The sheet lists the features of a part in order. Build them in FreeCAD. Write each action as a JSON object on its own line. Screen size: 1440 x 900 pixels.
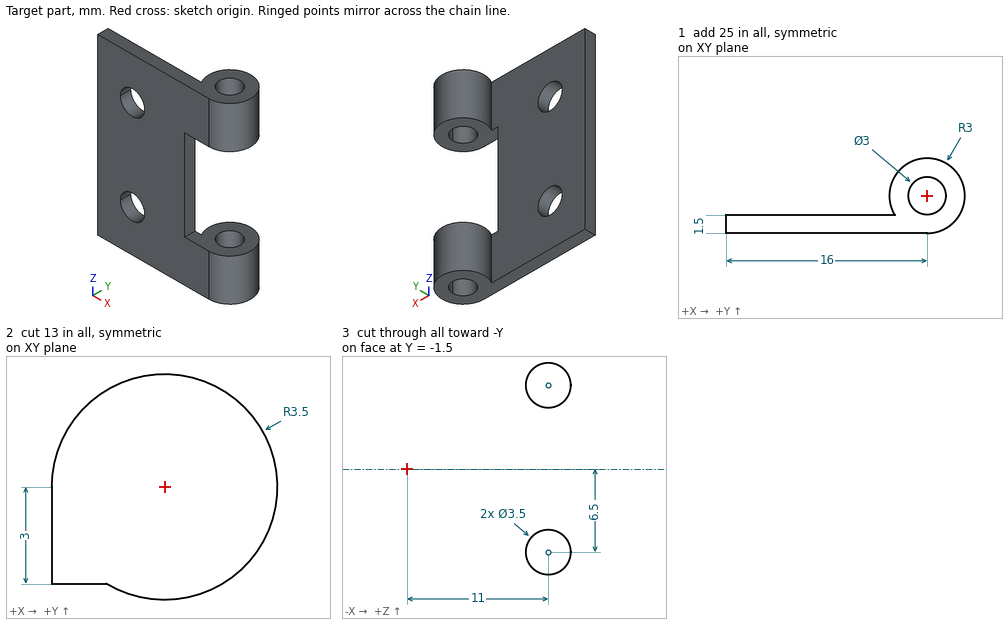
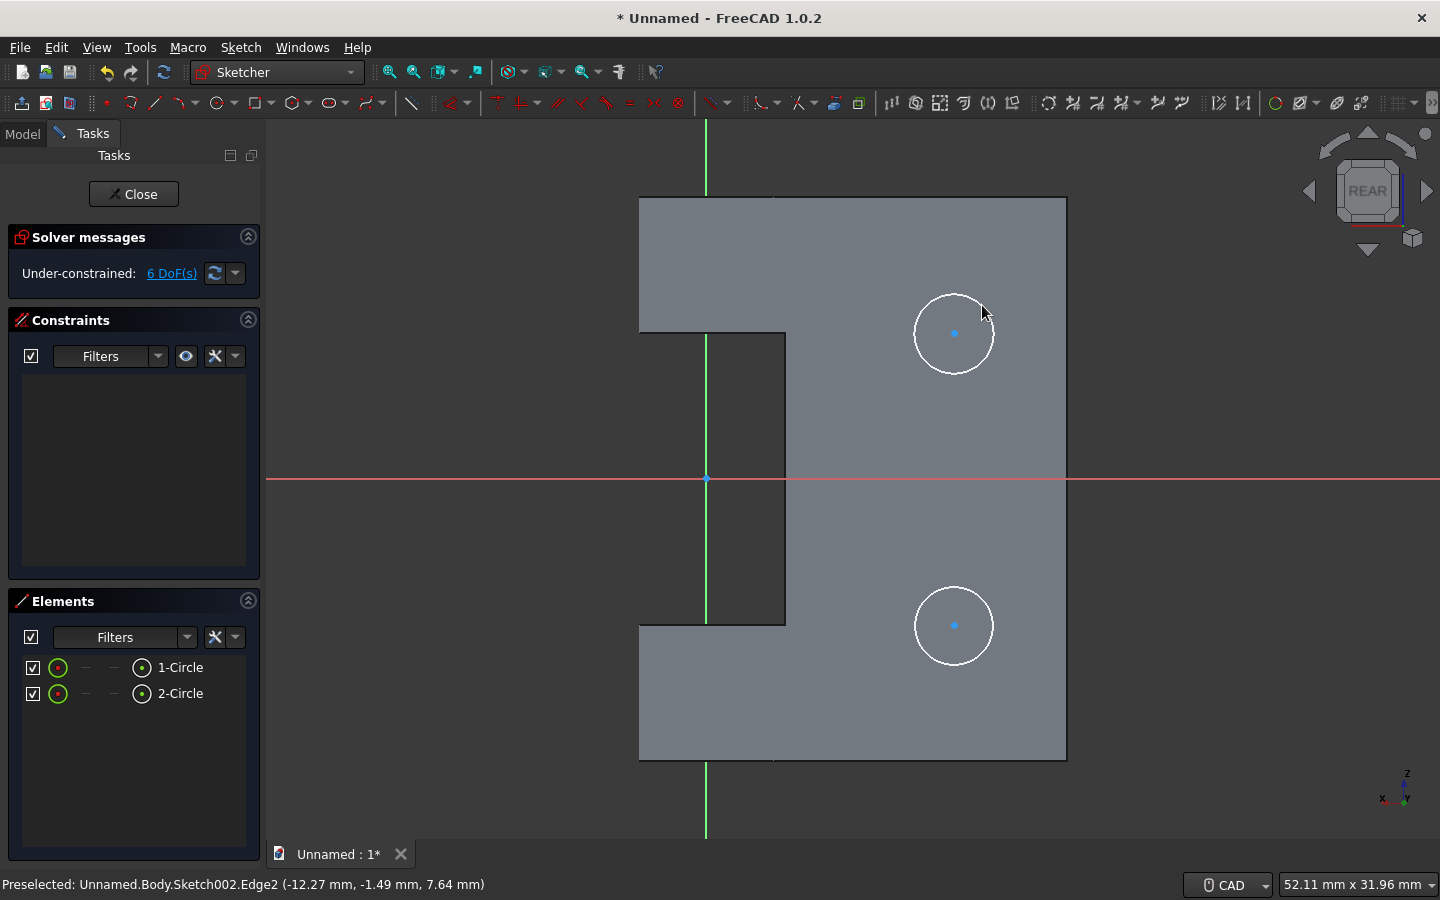
{"action": "left_click", "coordinate": [981, 598]}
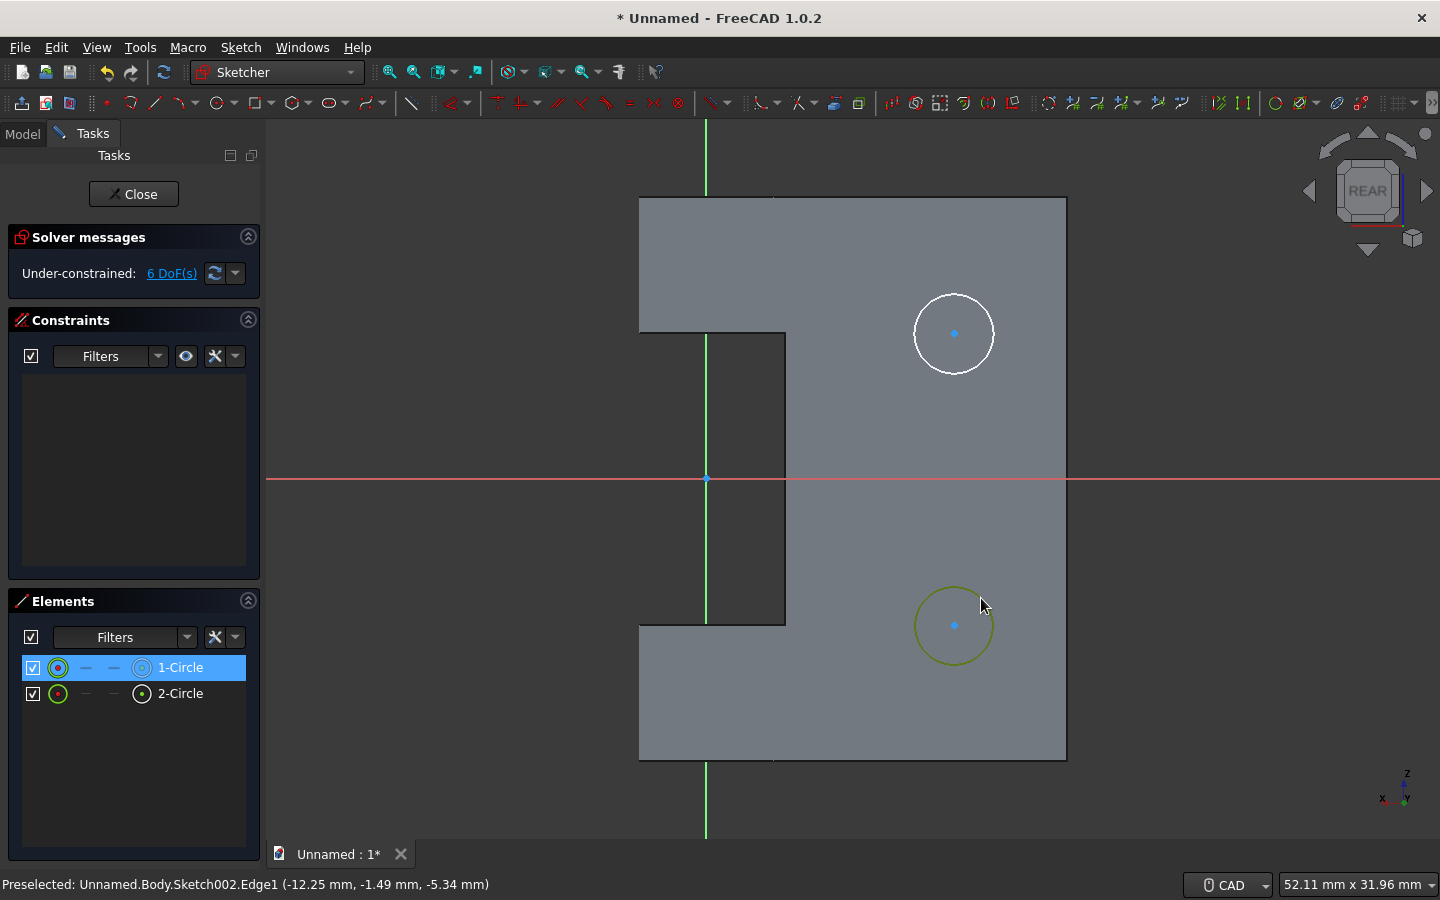
{"action": "left_click", "coordinate": [982, 306]}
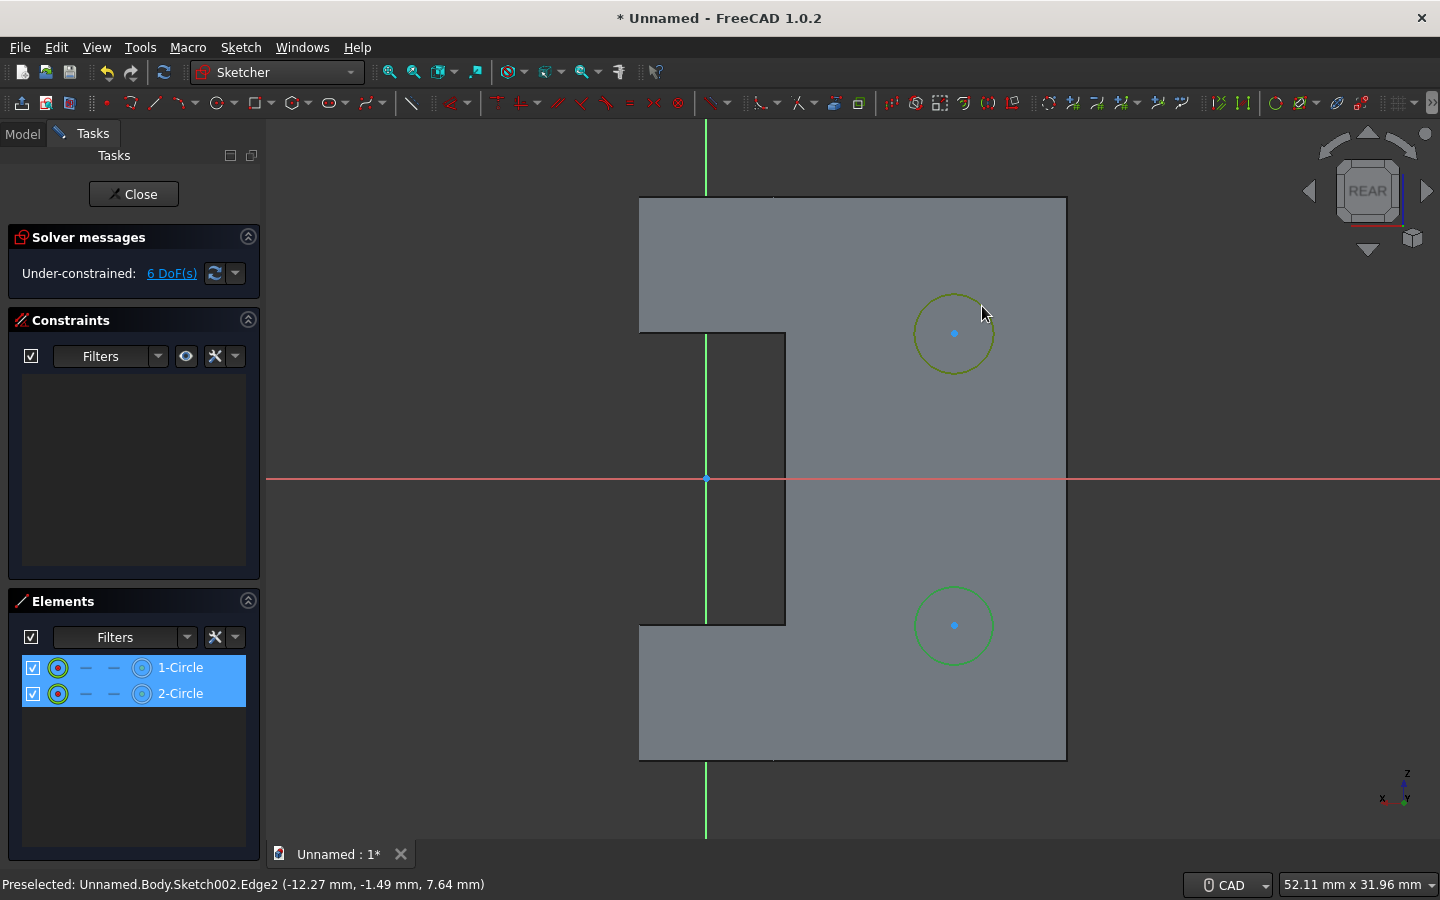
{"action": "left_click", "coordinate": [630, 104]}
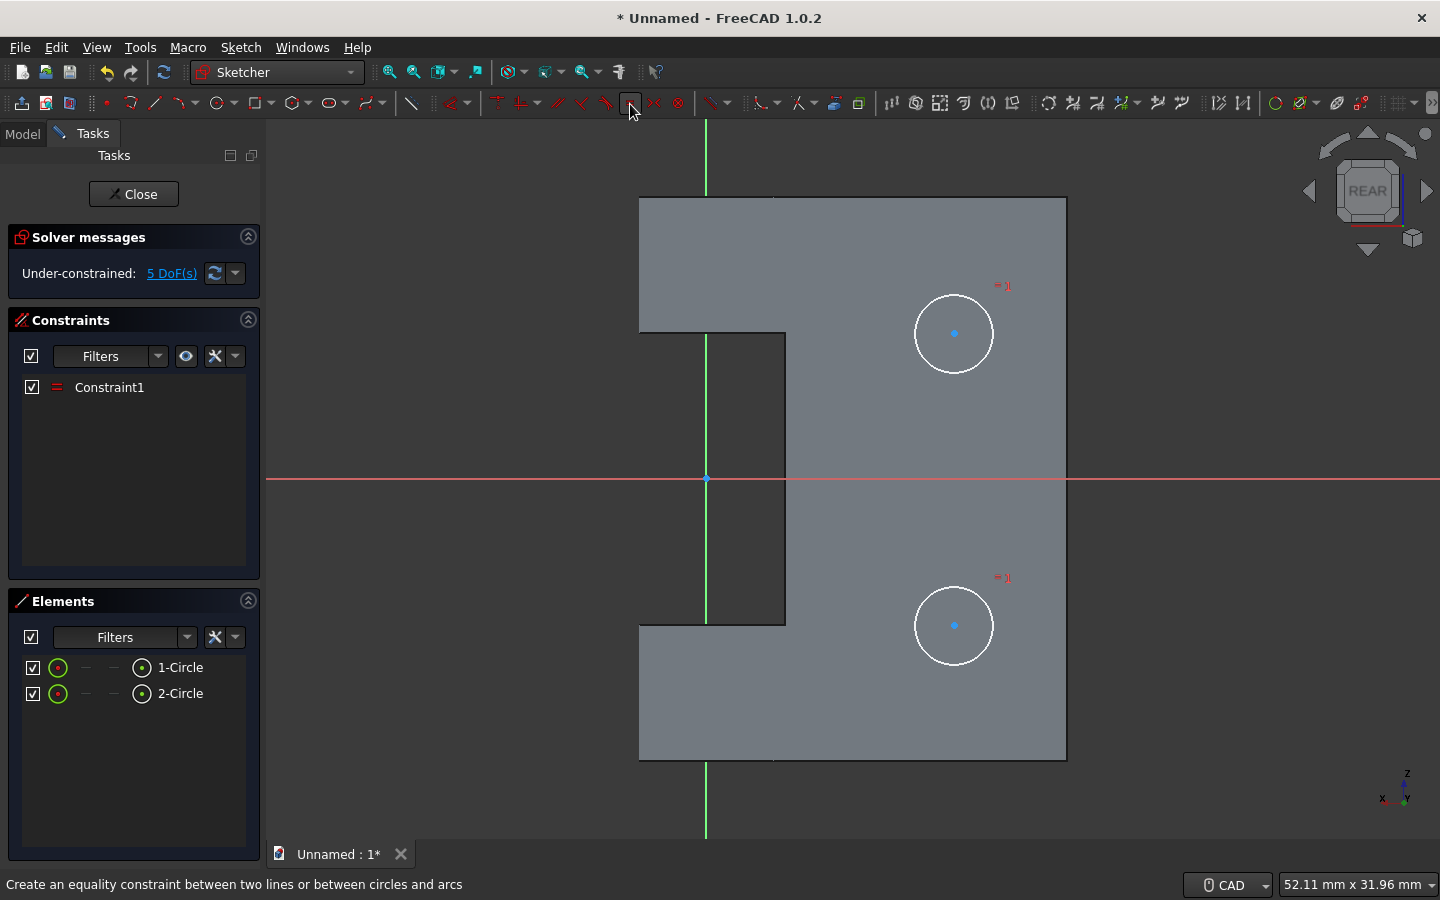
{"action": "left_click", "coordinate": [954, 626]}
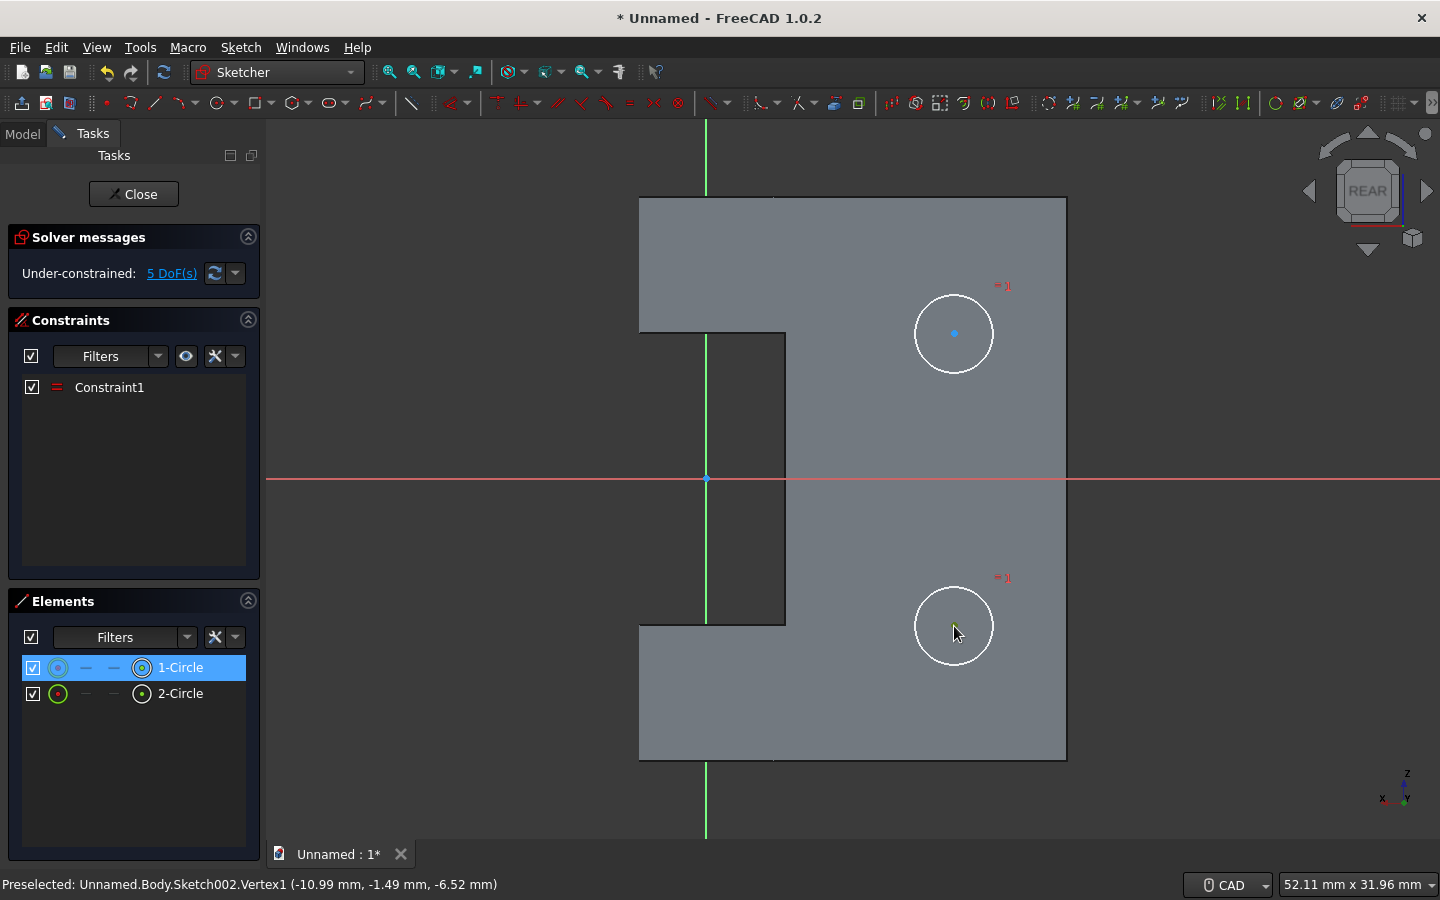
{"action": "left_click", "coordinate": [954, 334]}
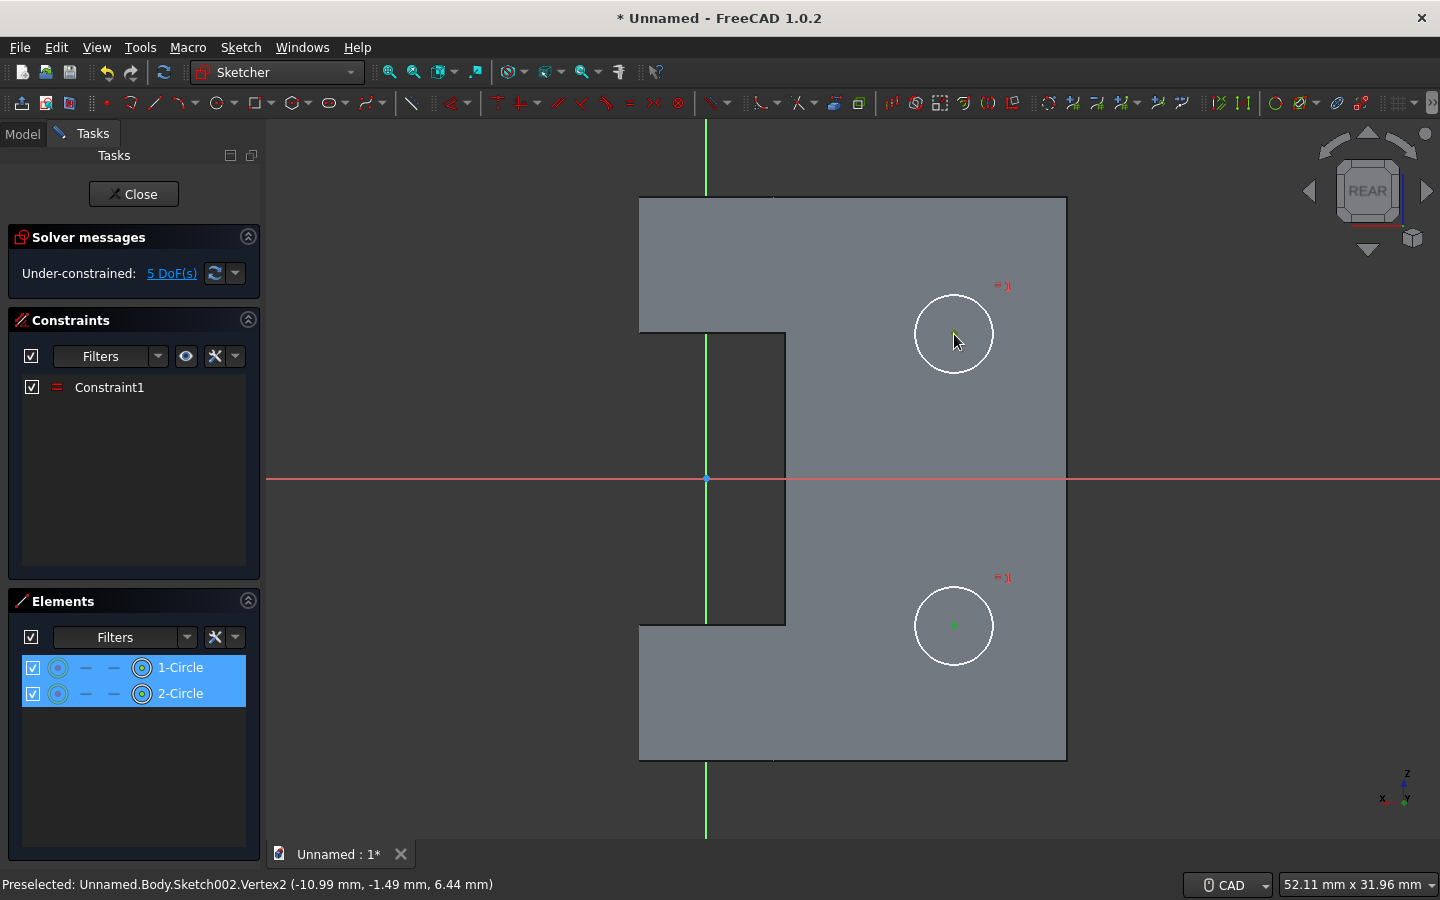
{"action": "left_click", "coordinate": [364, 479]}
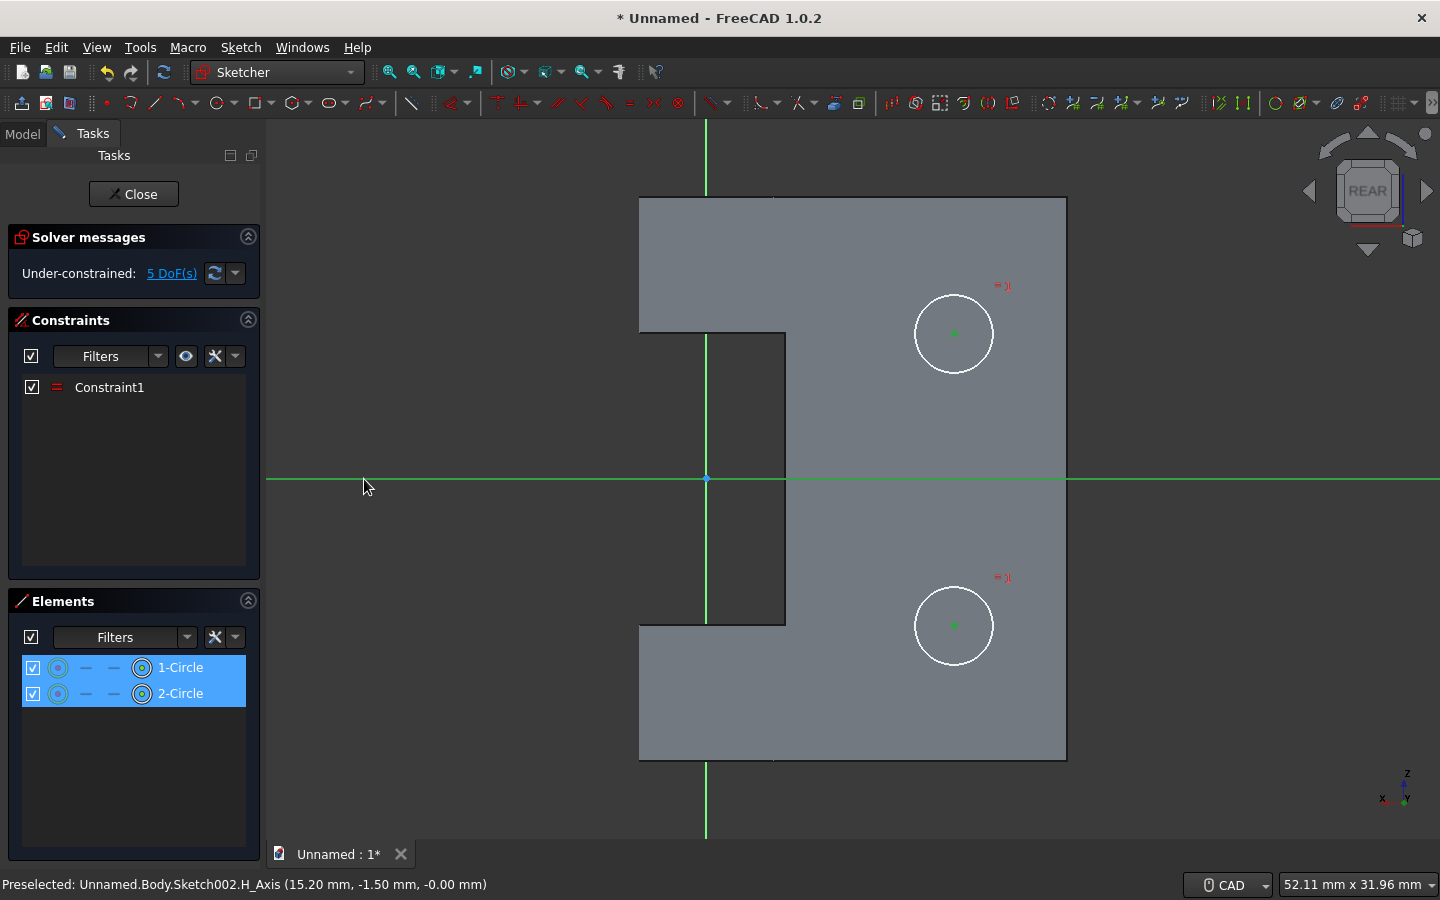
{"action": "left_click", "coordinate": [654, 104]}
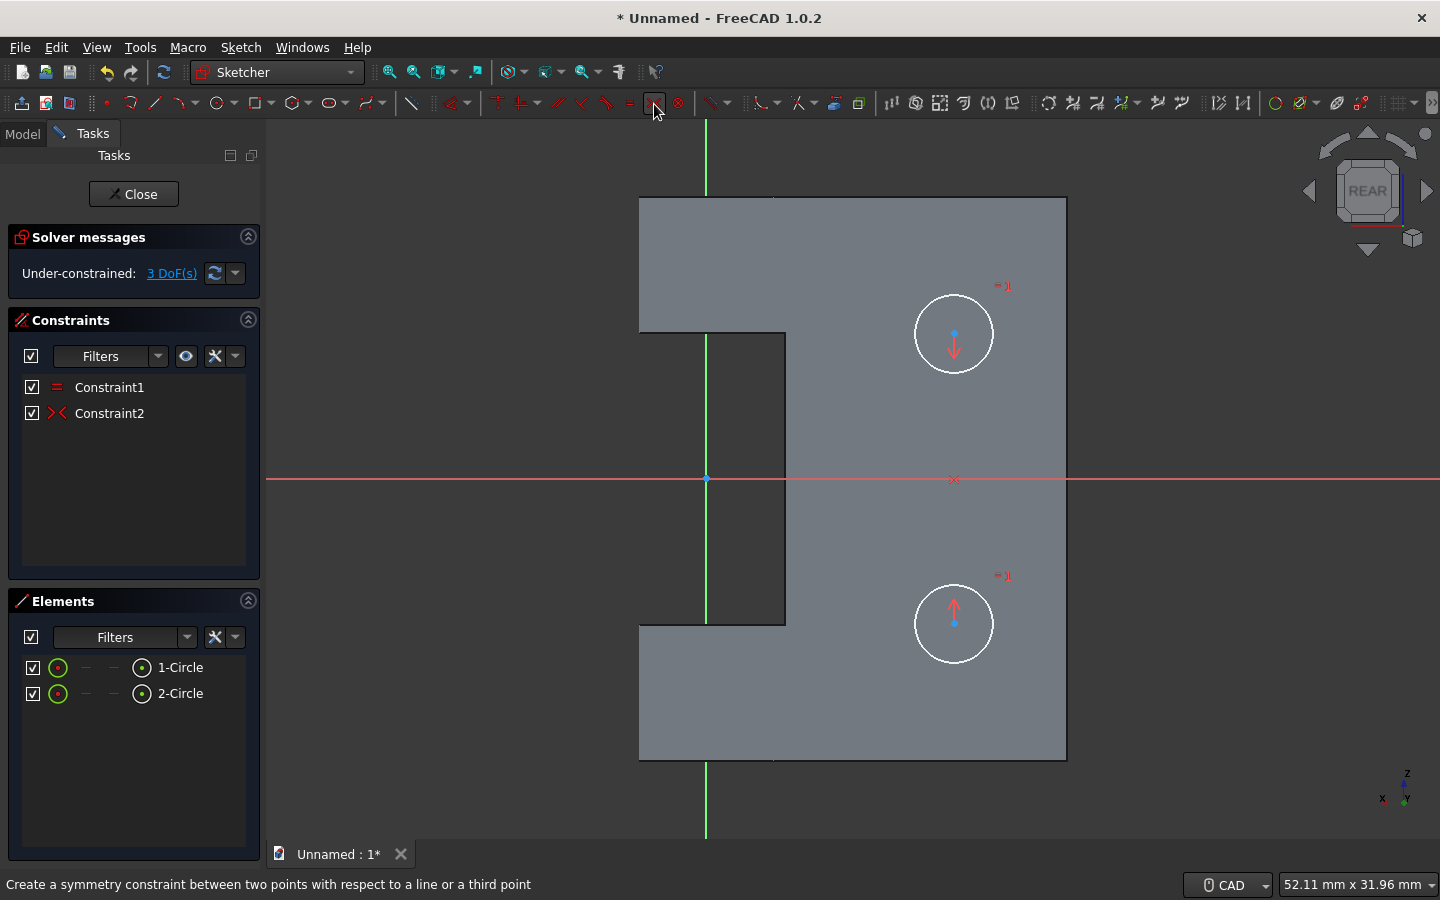
{"action": "left_click", "coordinate": [450, 104]}